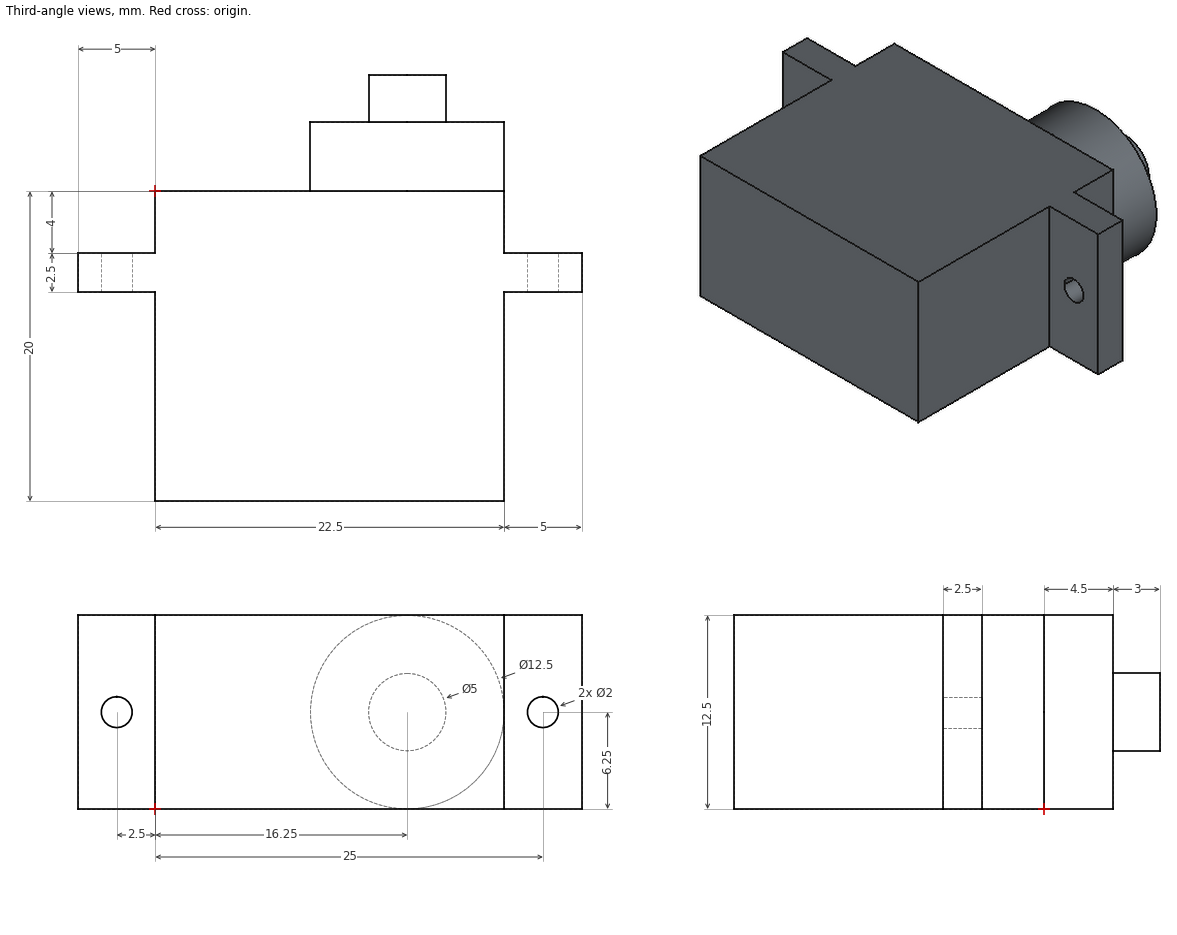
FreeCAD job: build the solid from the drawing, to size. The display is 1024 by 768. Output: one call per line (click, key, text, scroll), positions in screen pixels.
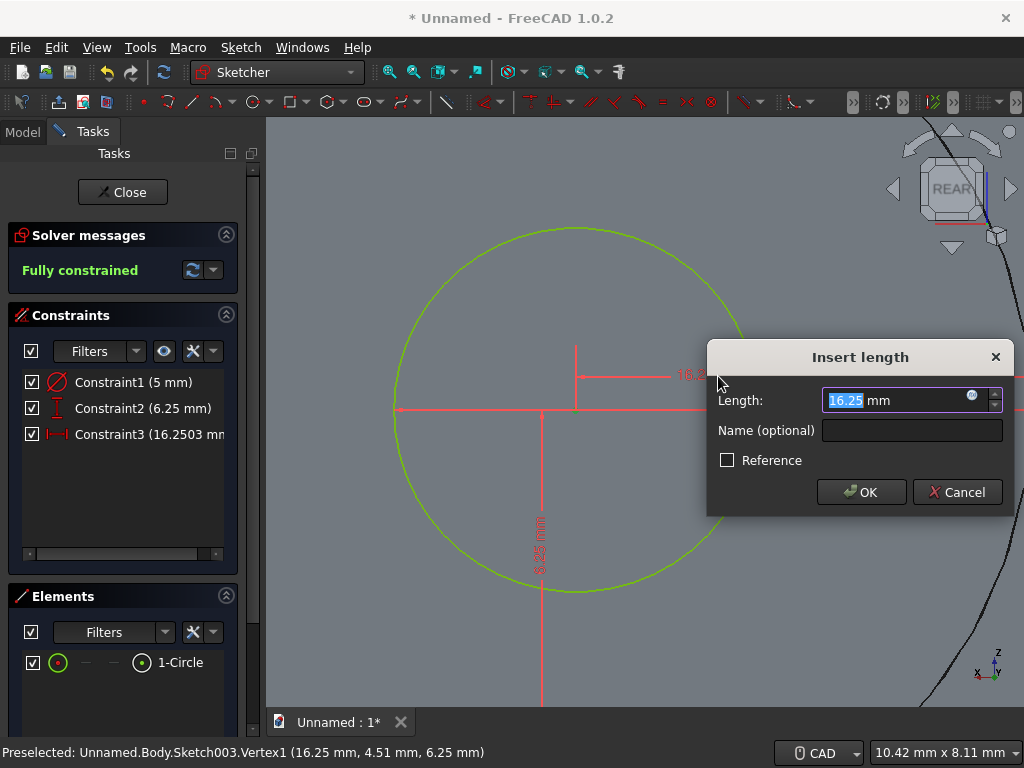
text(16.25)
key(Return)
key(Escape)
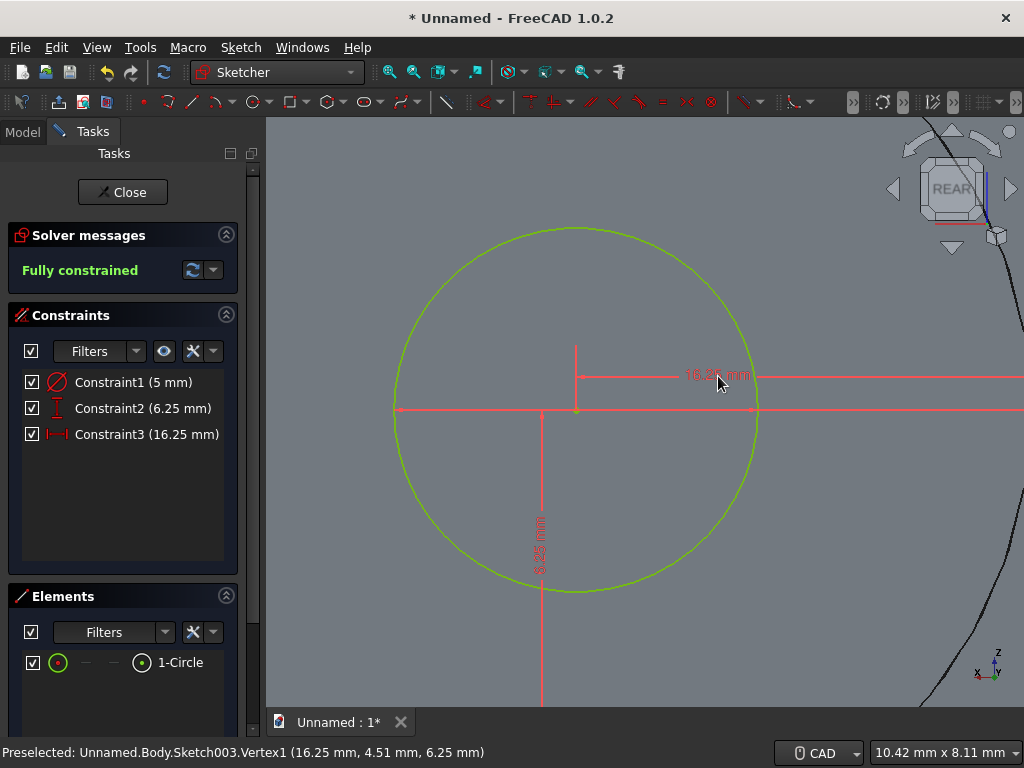
click(123, 192)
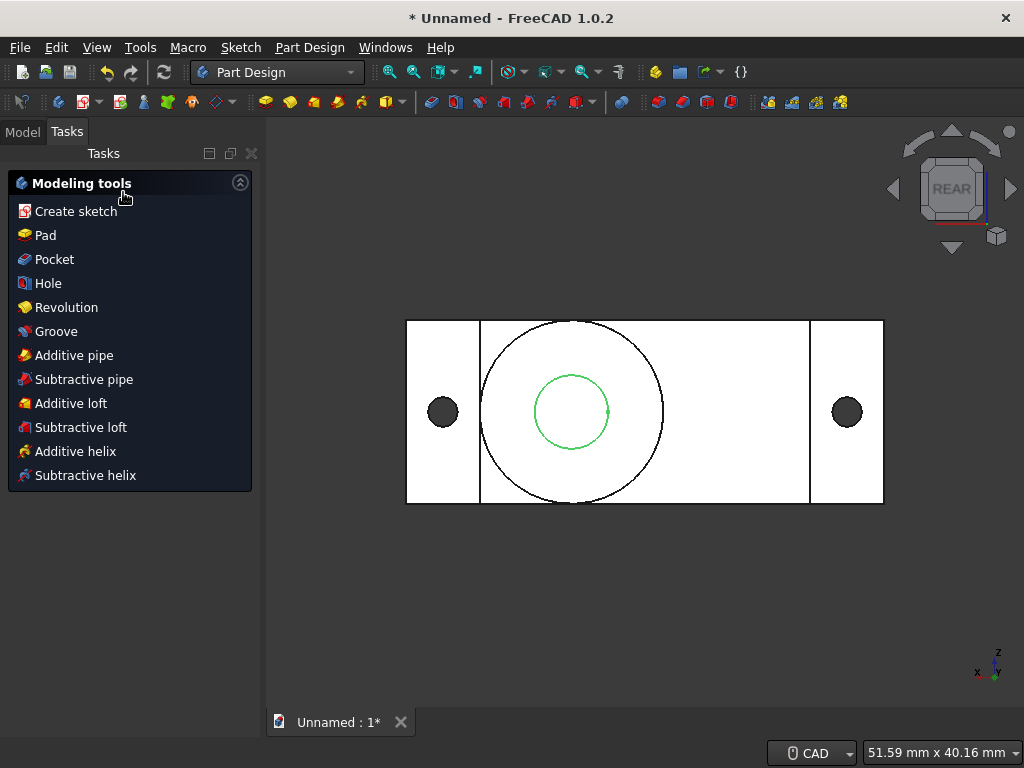
click(266, 102)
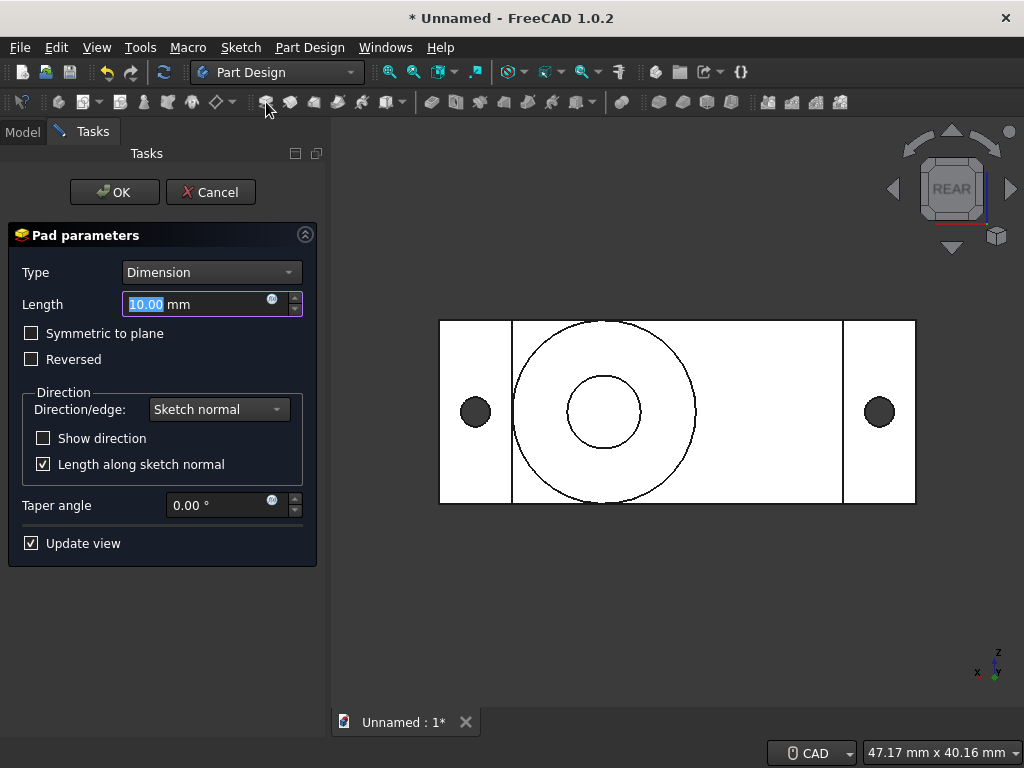
text(3)
key(Tab)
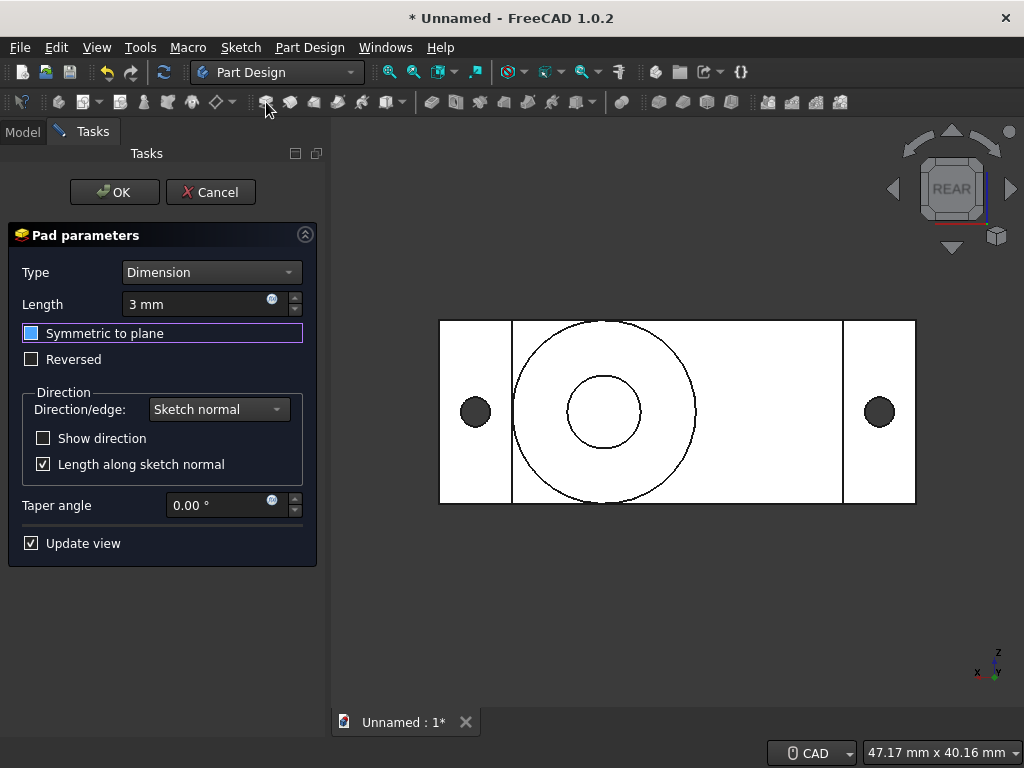
click(115, 192)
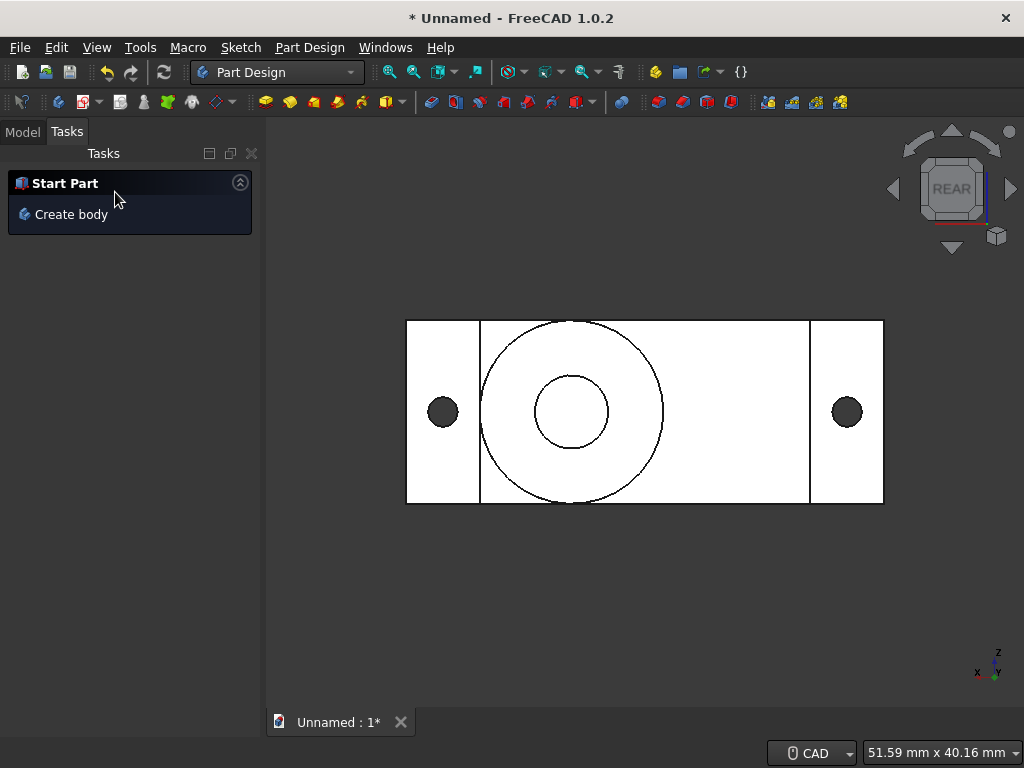
key(0)